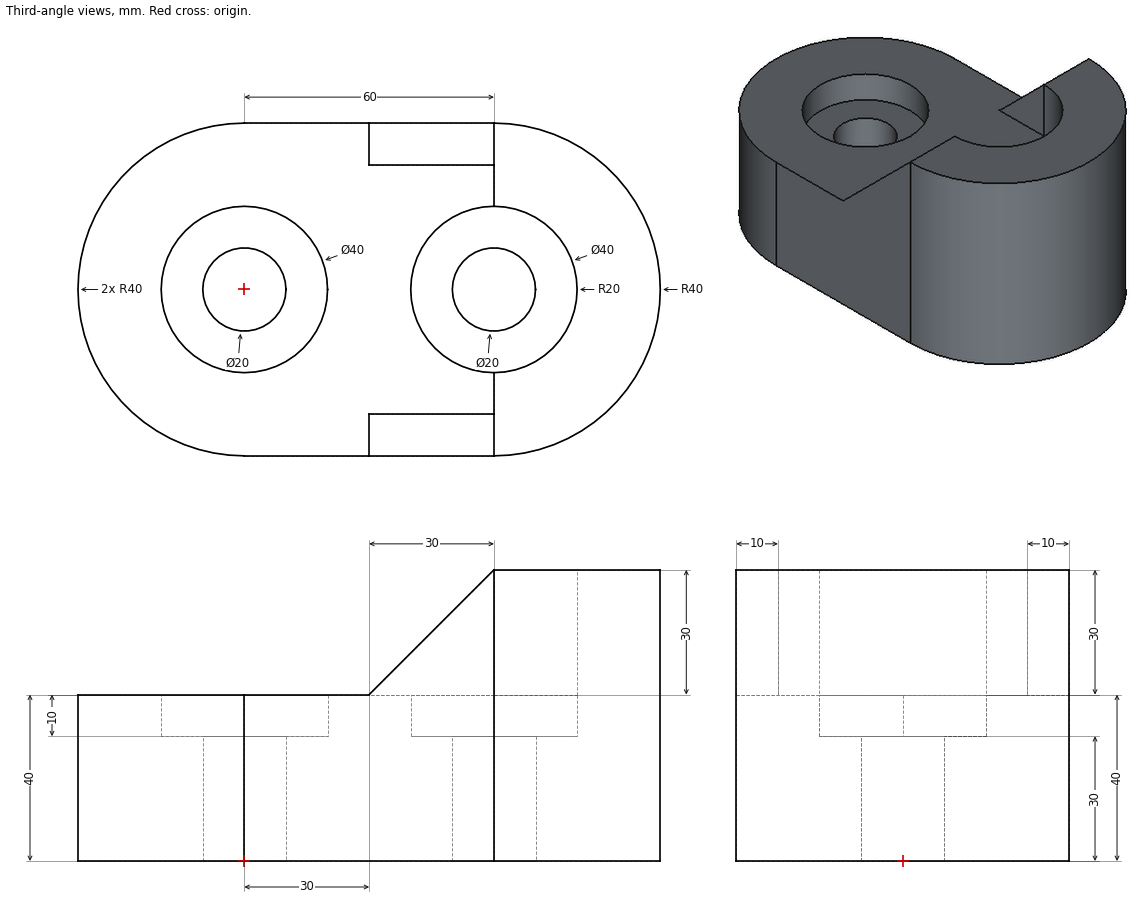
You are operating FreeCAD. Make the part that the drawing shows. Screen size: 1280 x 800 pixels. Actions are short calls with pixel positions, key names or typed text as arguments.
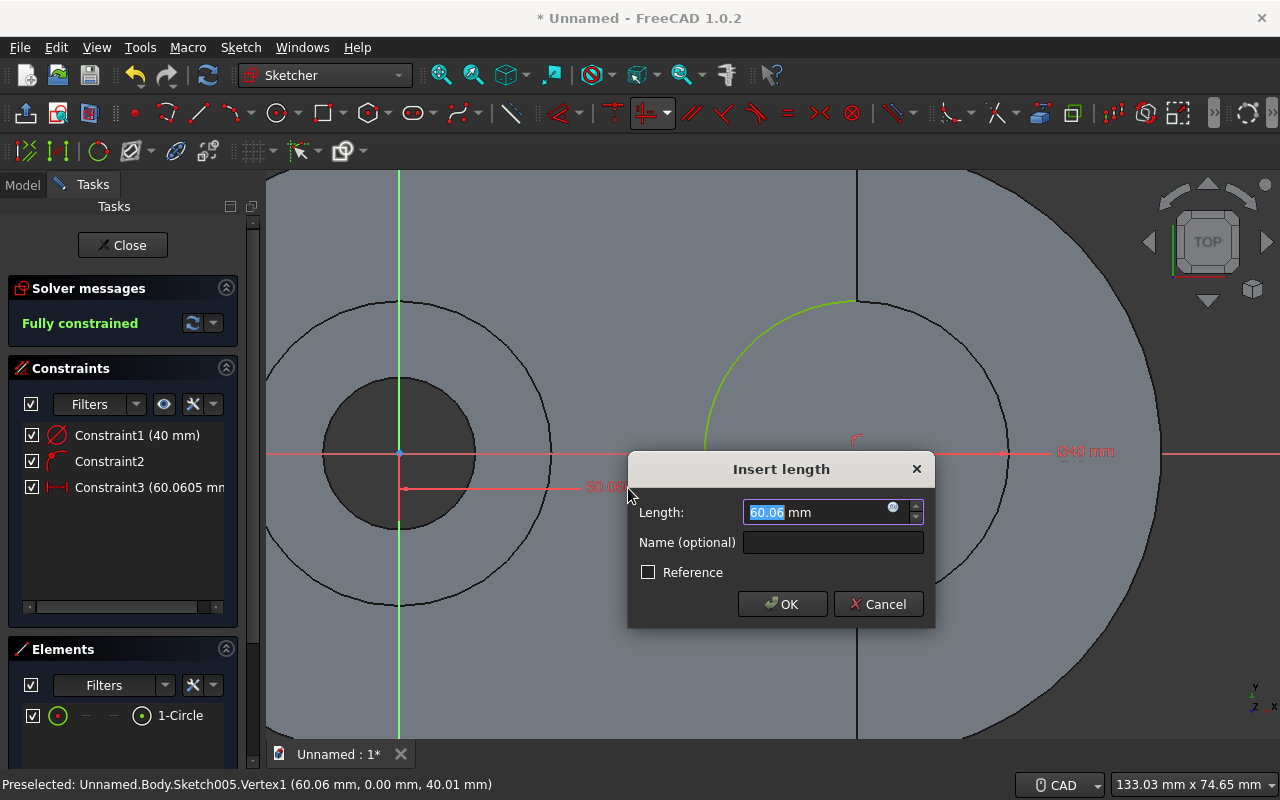
text(60)
key(Return)
key(Escape)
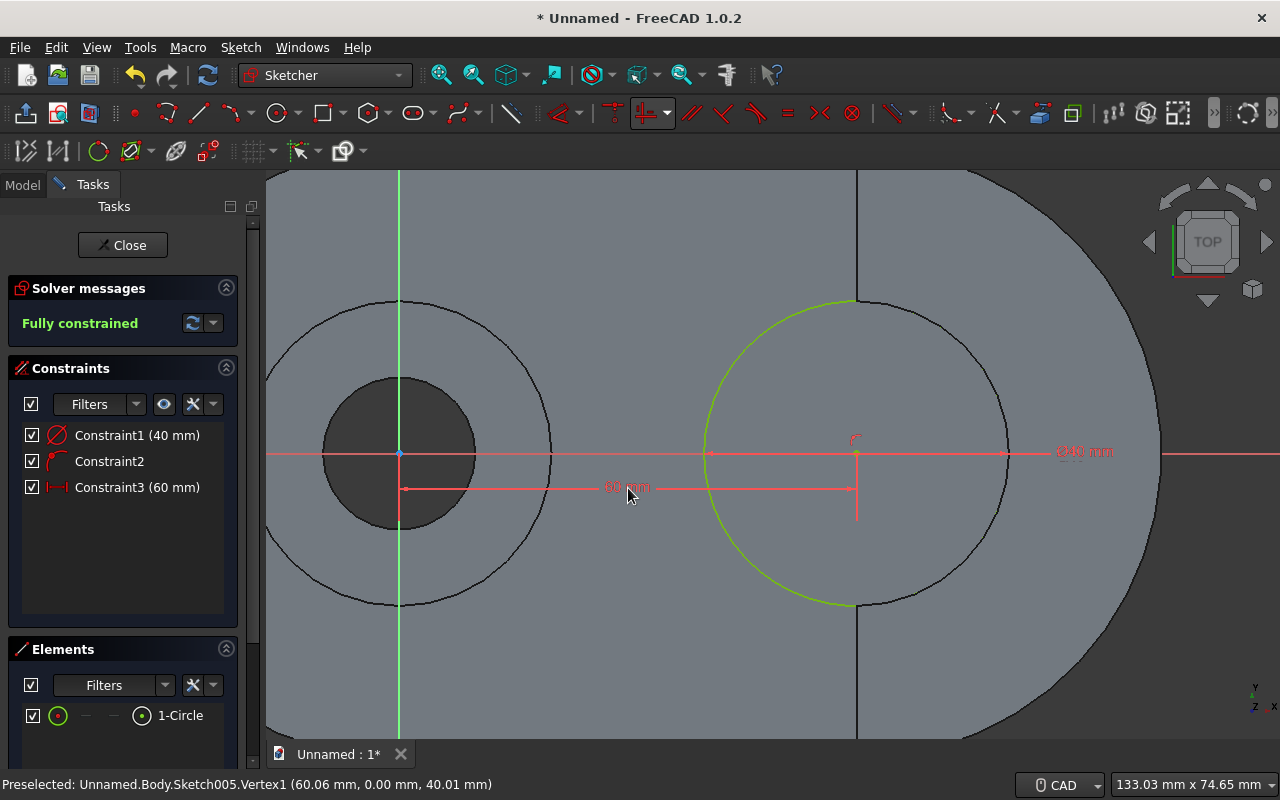
click(123, 245)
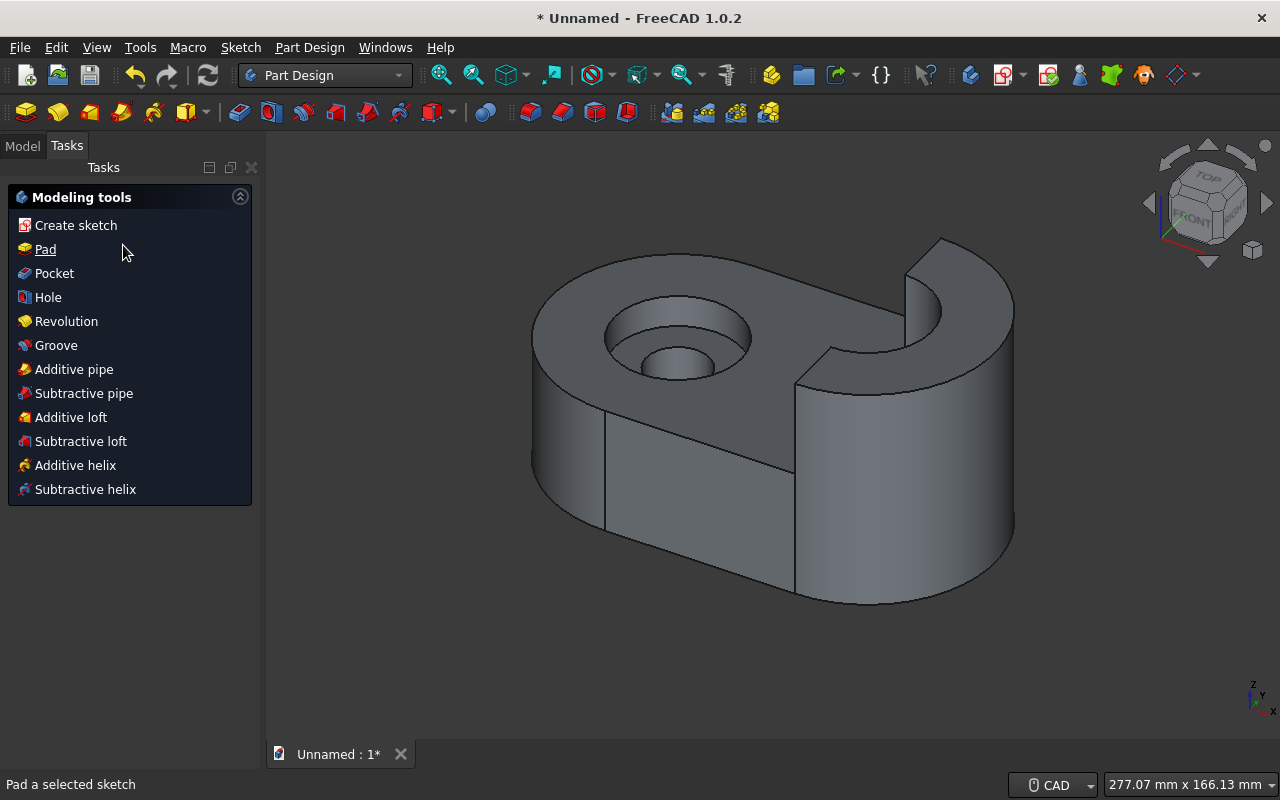
click(240, 112)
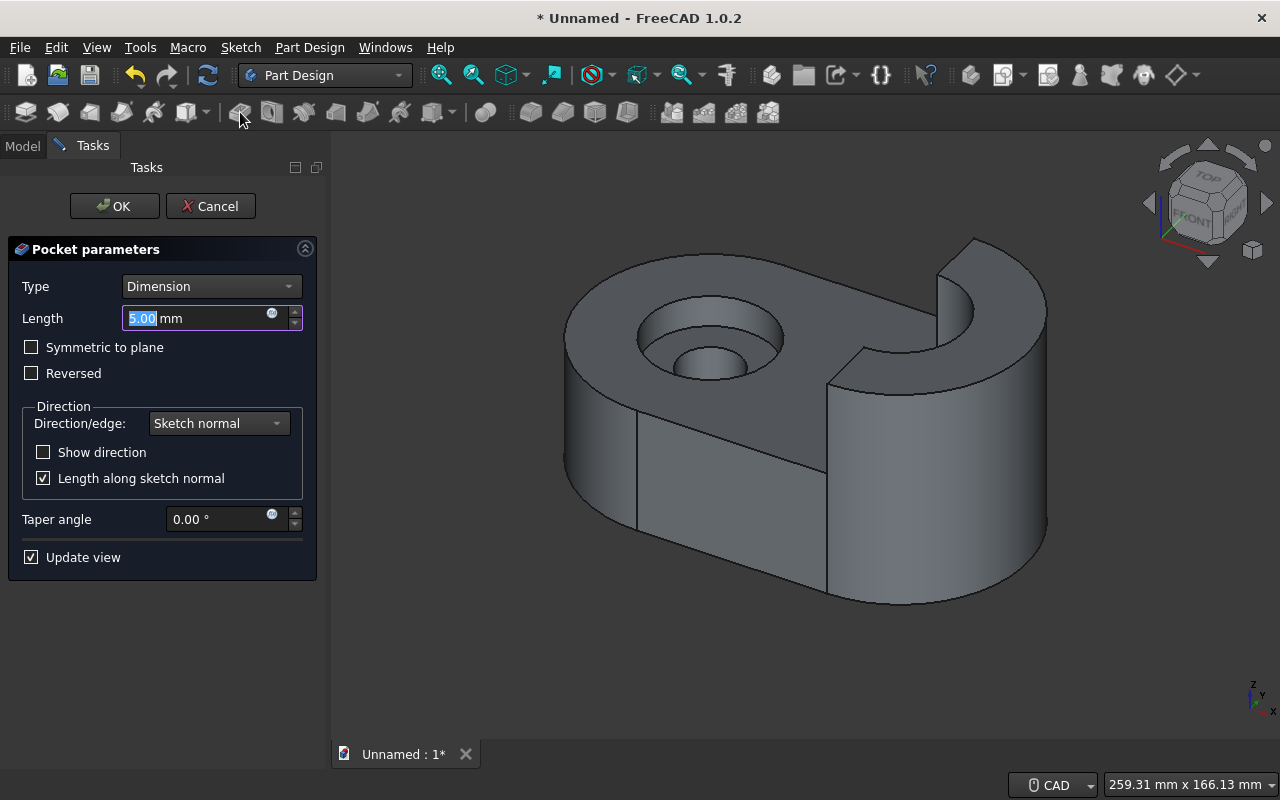
text(10)
key(Tab)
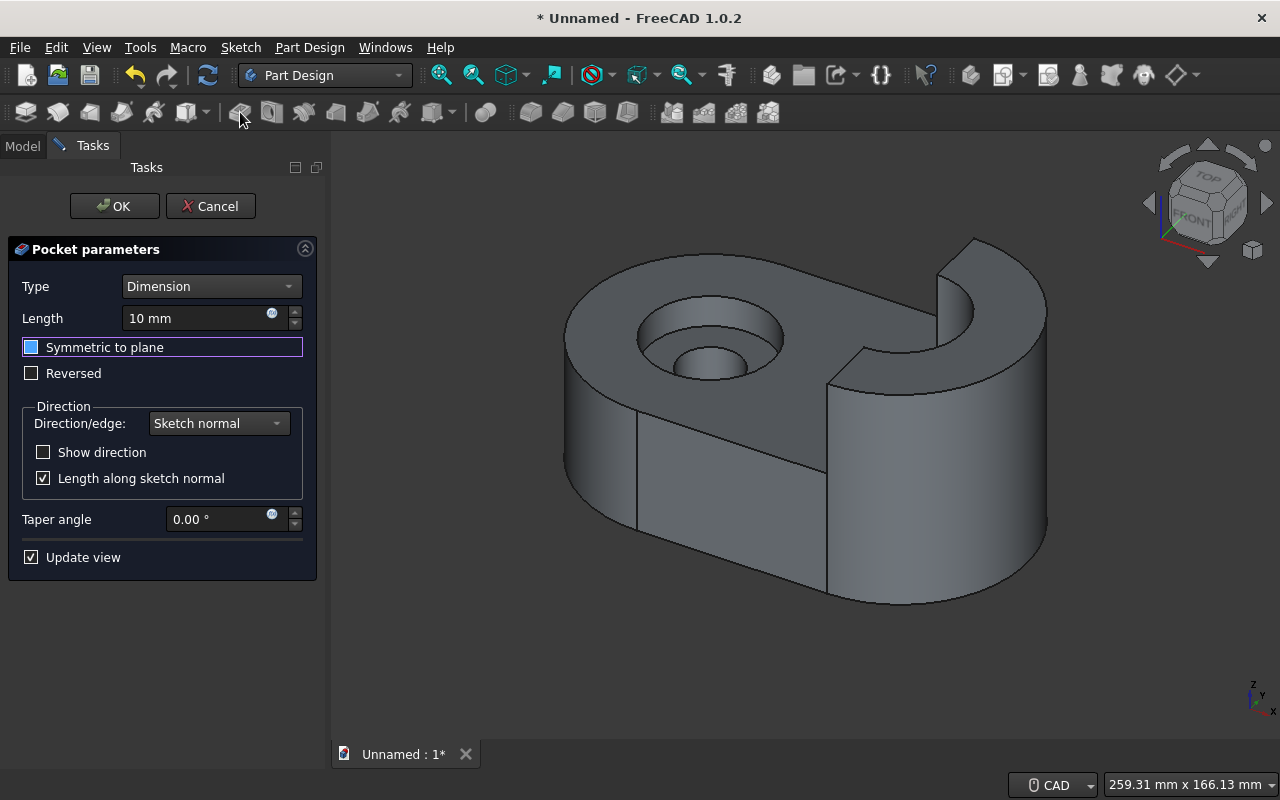
click(115, 206)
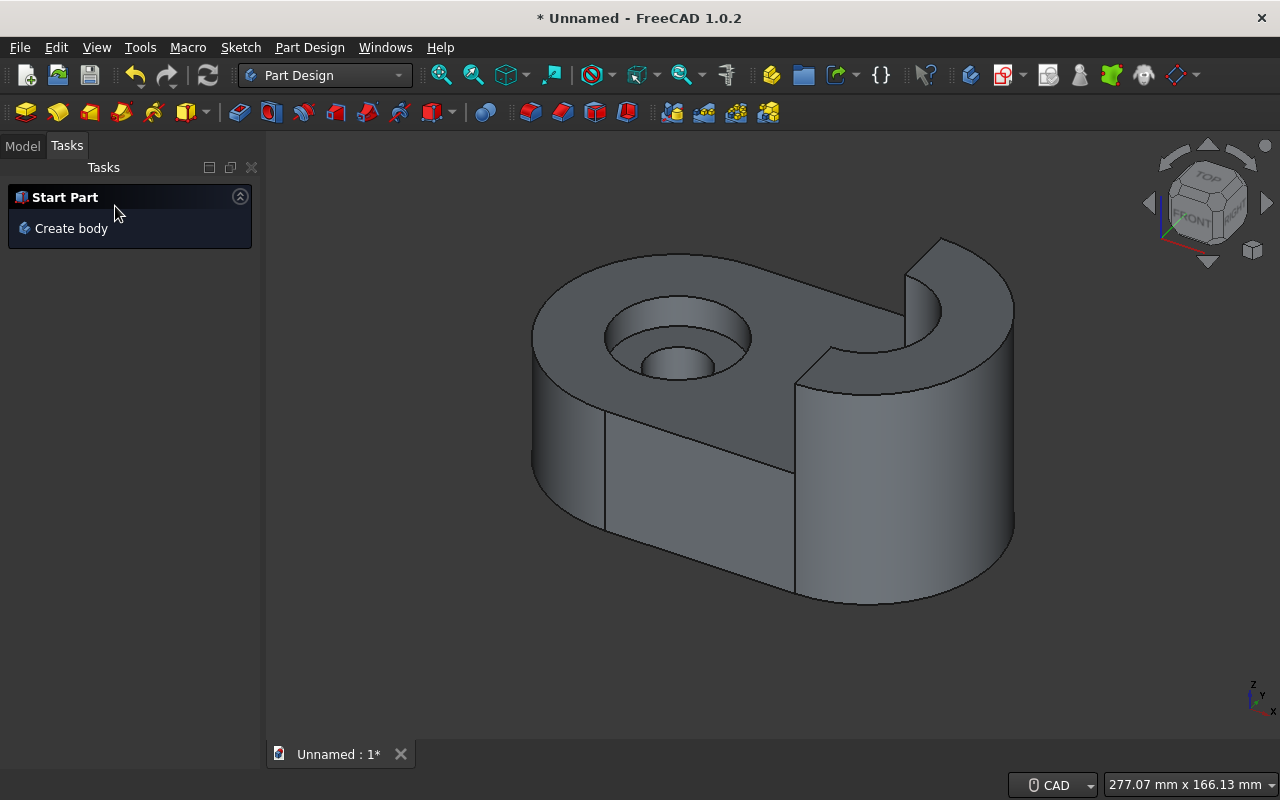
key(0)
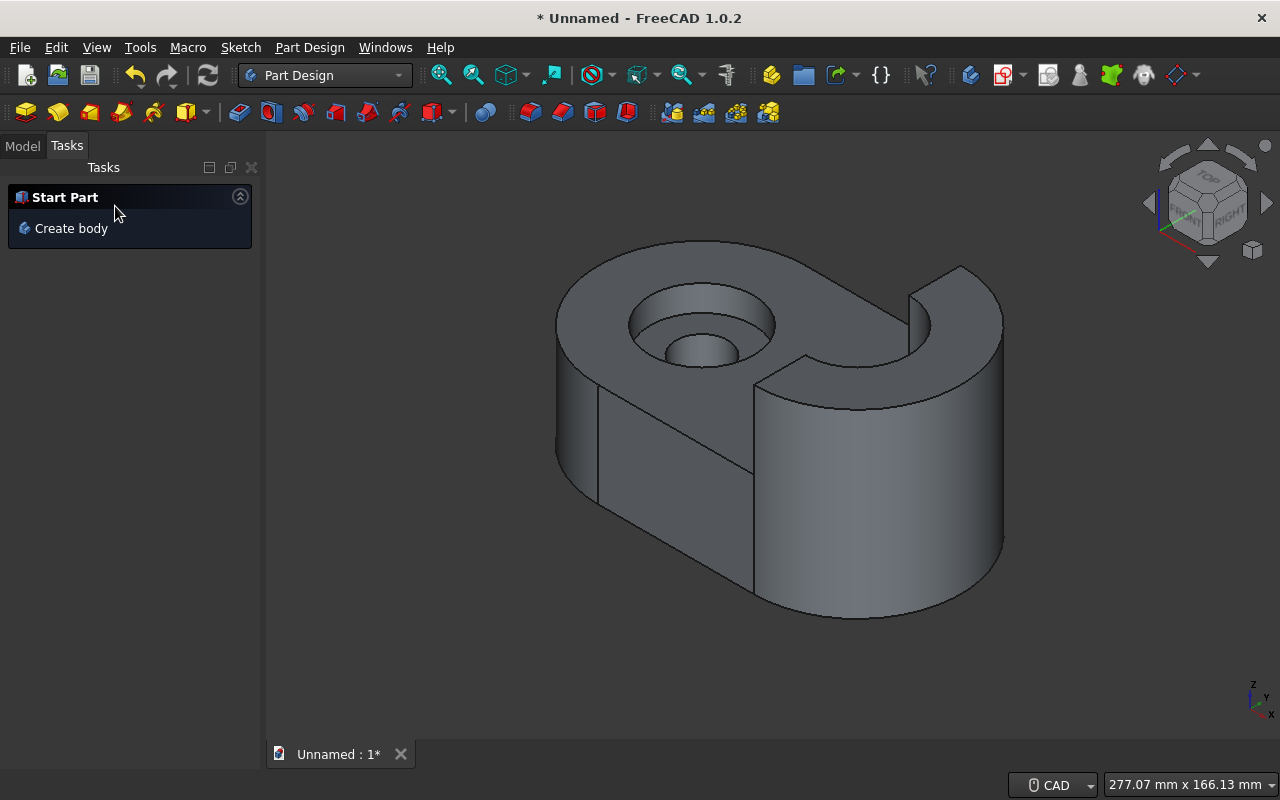
click(442, 76)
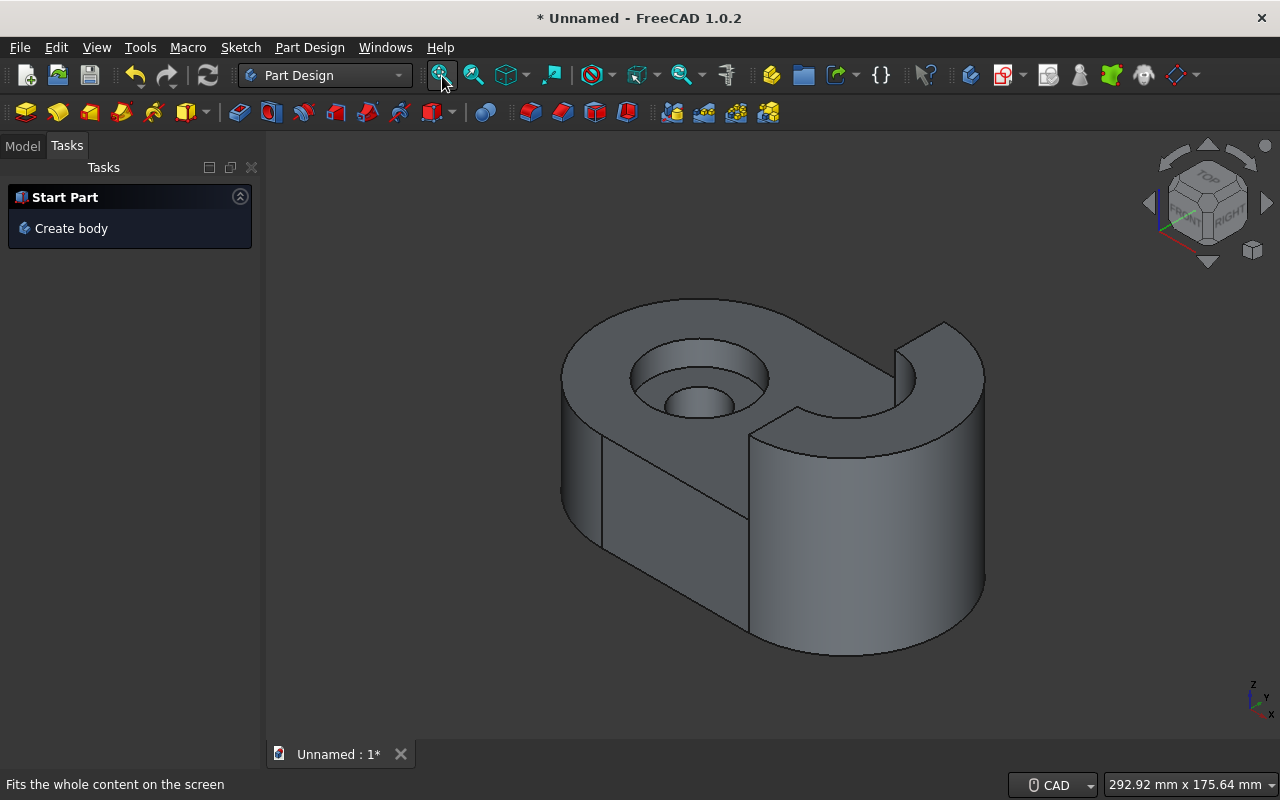
key(2)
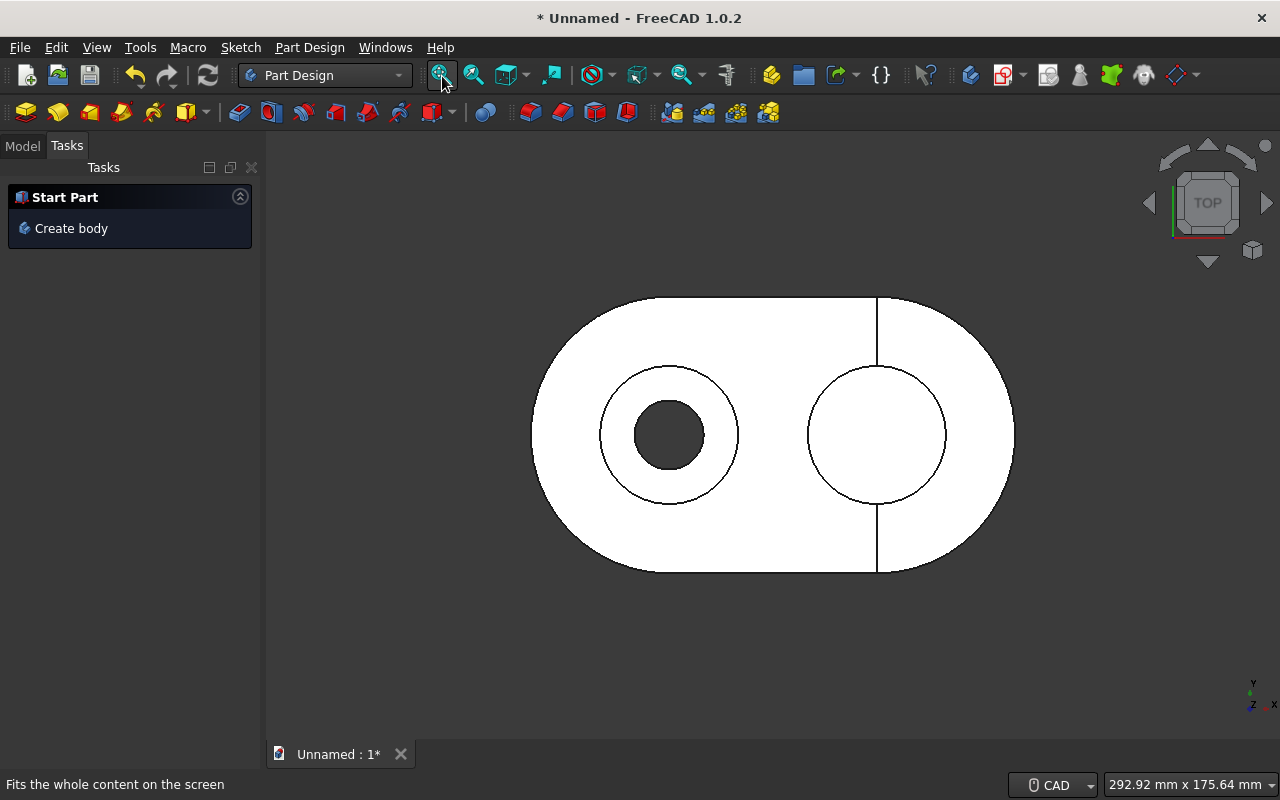
click(877, 434)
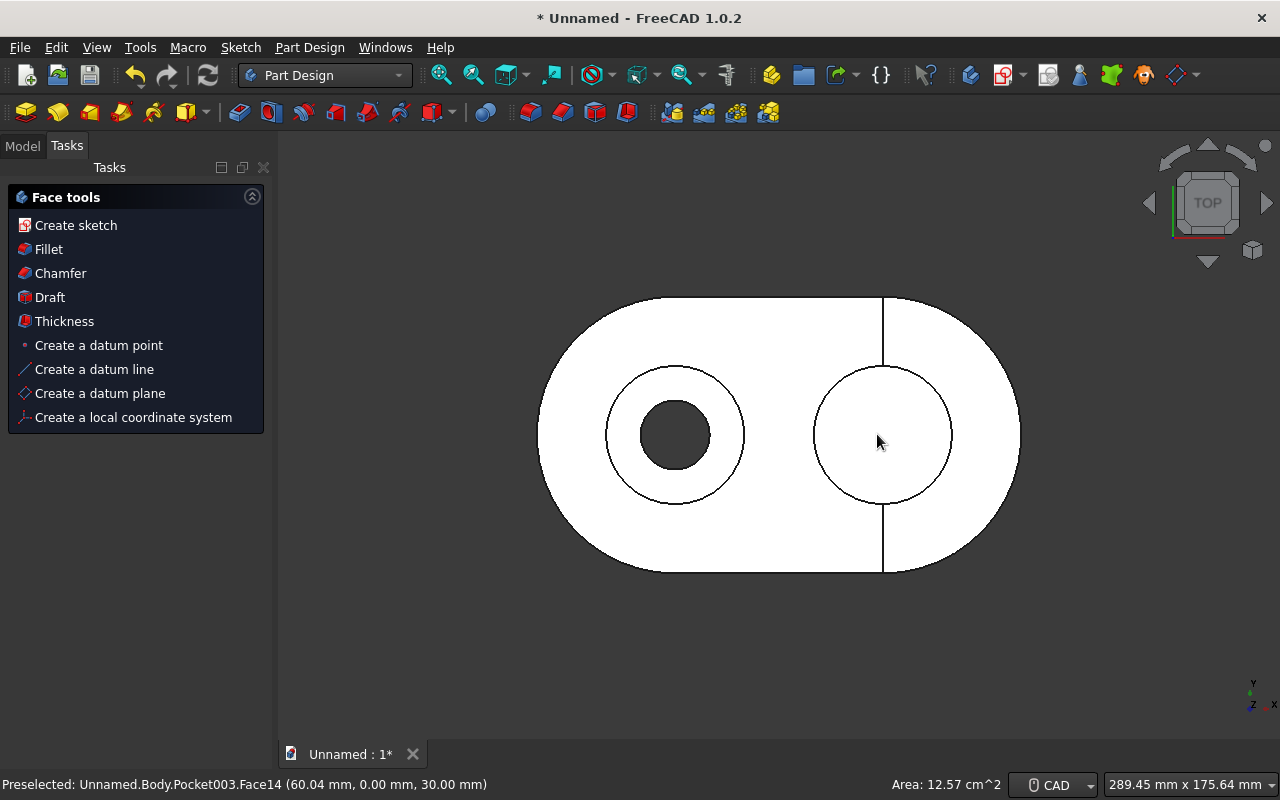
click(1004, 76)